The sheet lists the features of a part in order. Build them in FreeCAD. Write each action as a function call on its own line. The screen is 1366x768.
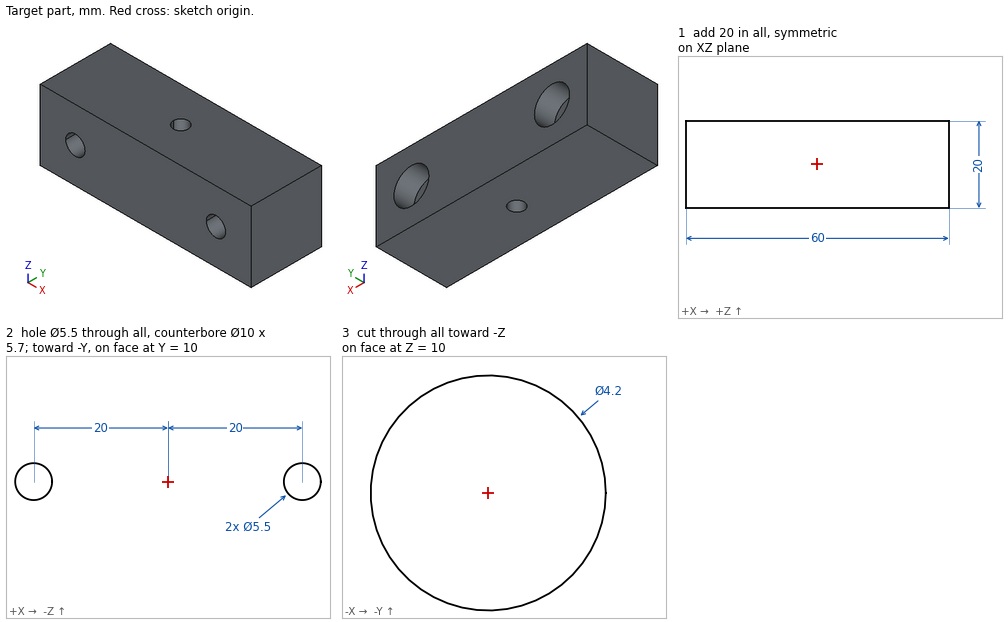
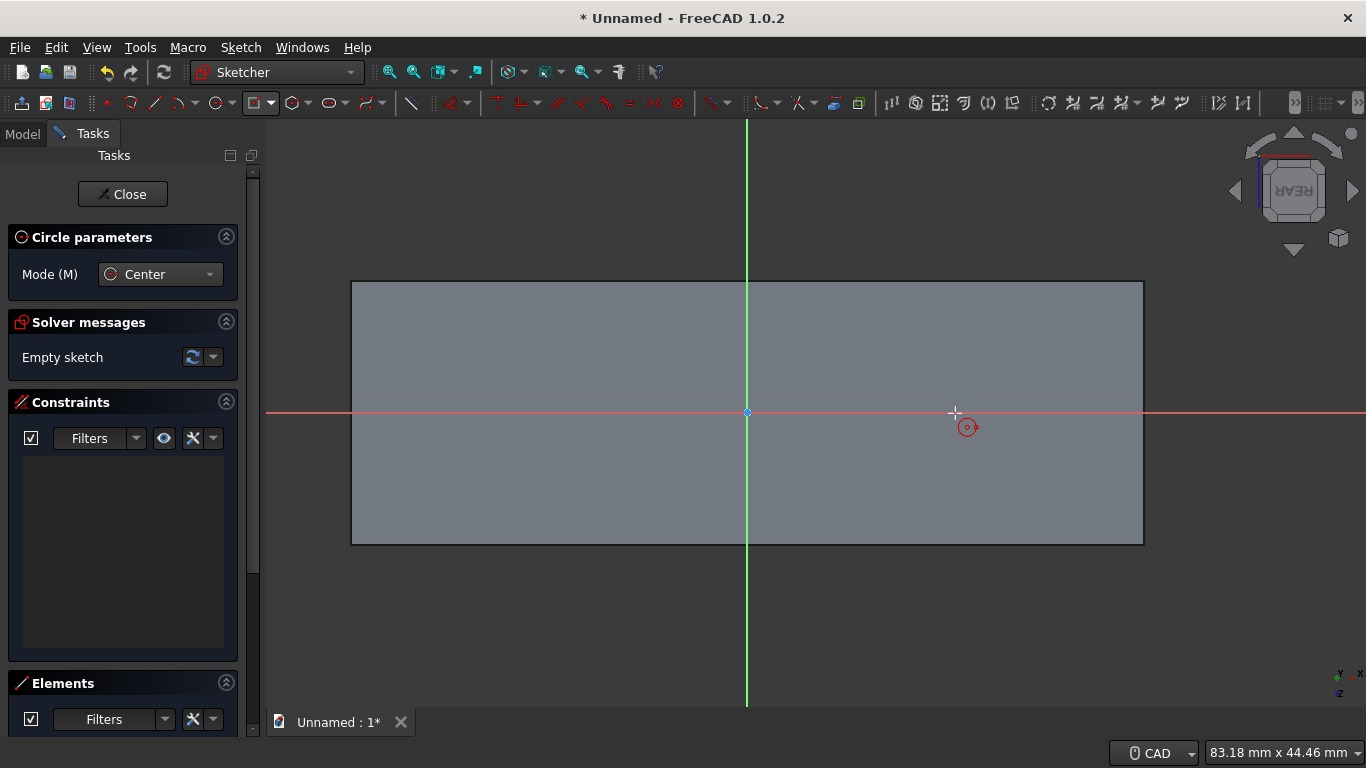
click(1012, 413)
move(1038, 387)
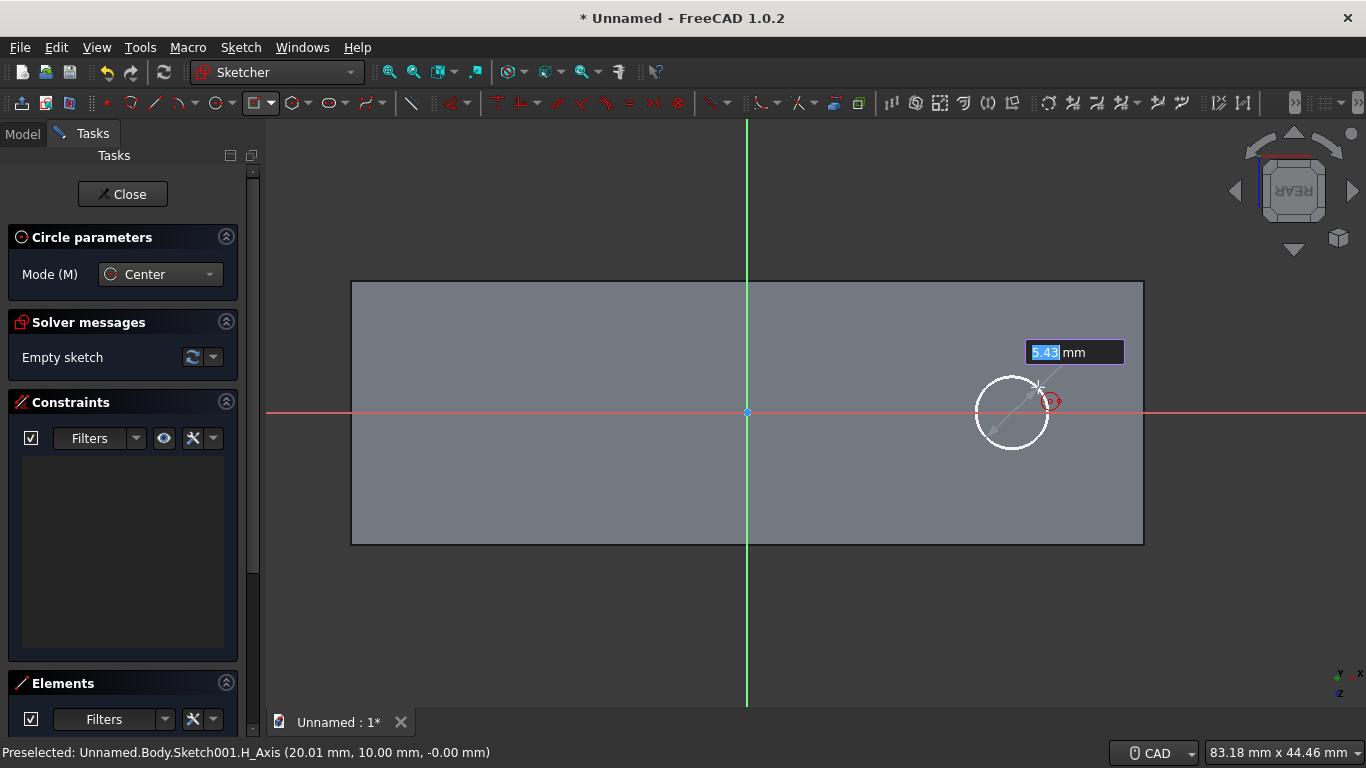
text(5.5)
key(Return)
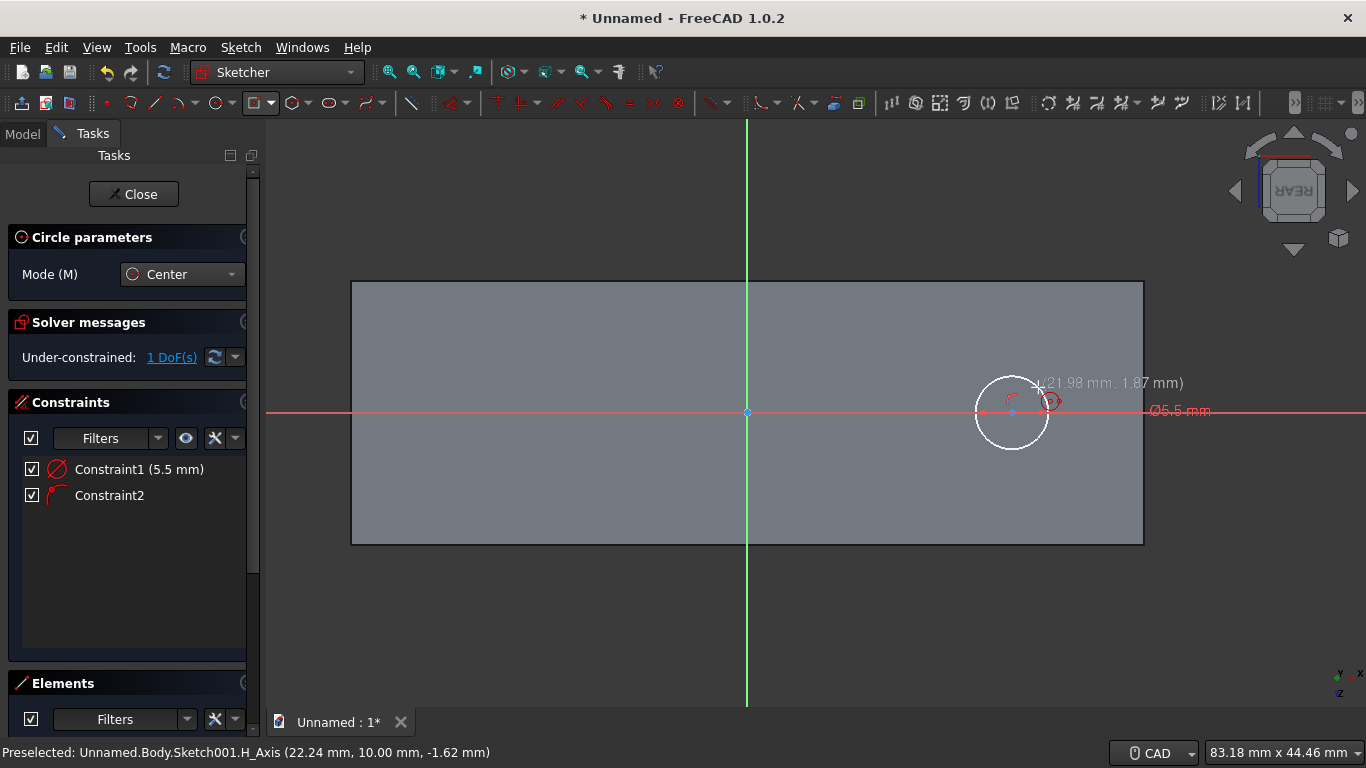
click(483, 413)
move(509, 387)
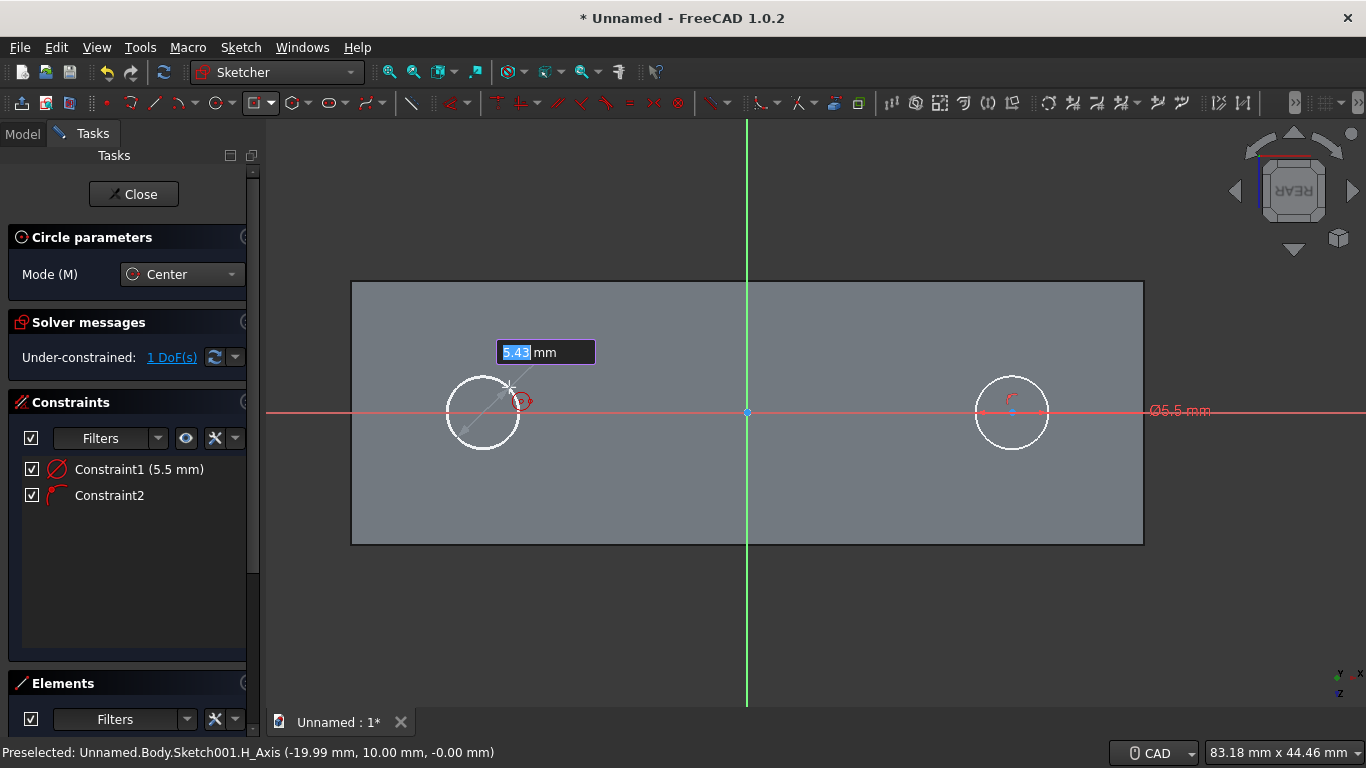
text(5.5)
key(Return)
key(Escape)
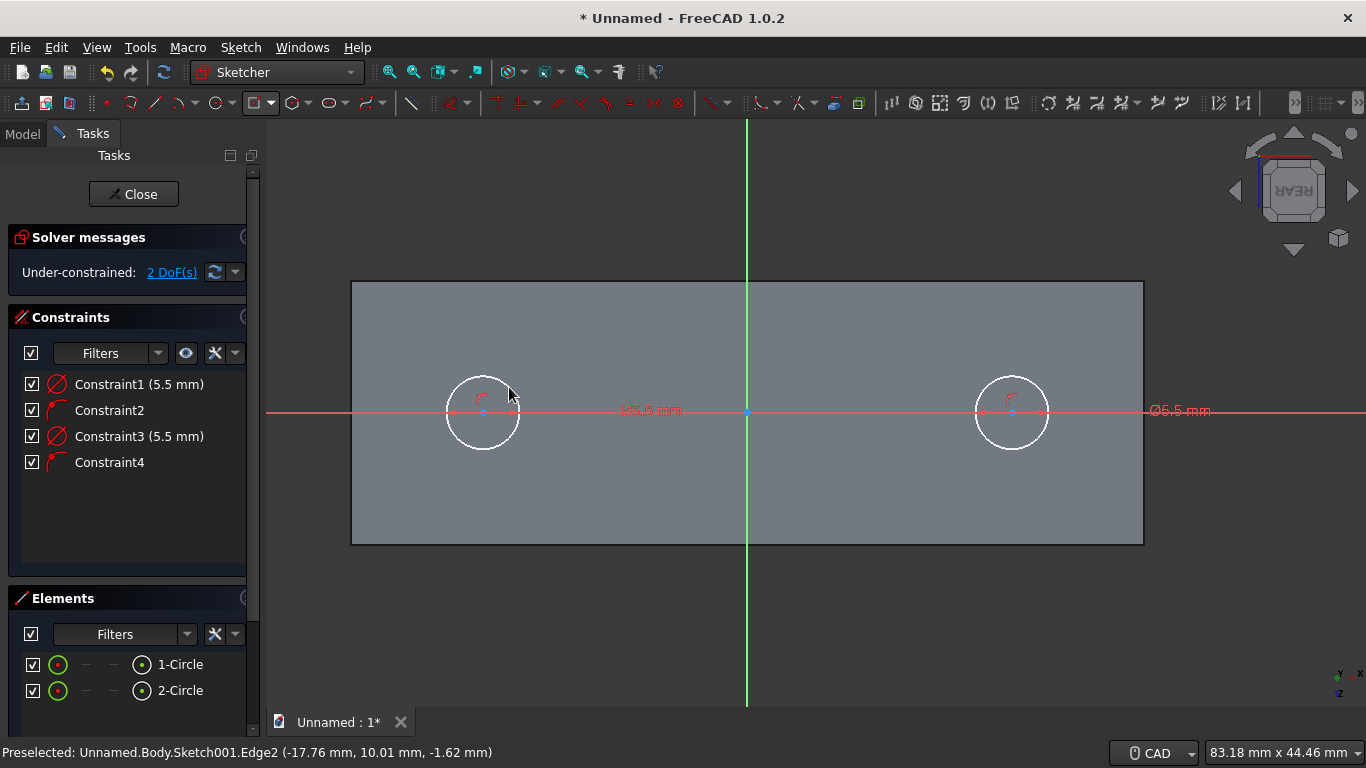
key(d)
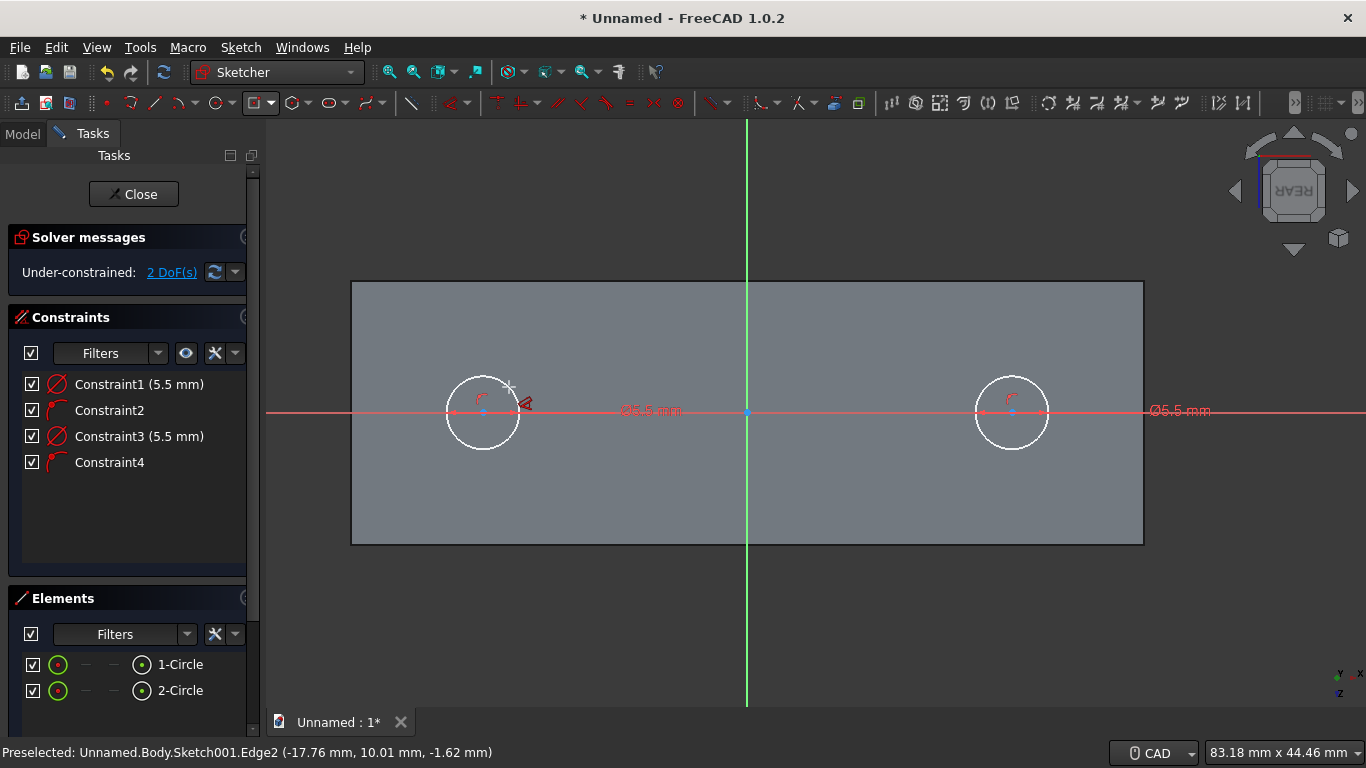
click(1012, 413)
click(880, 447)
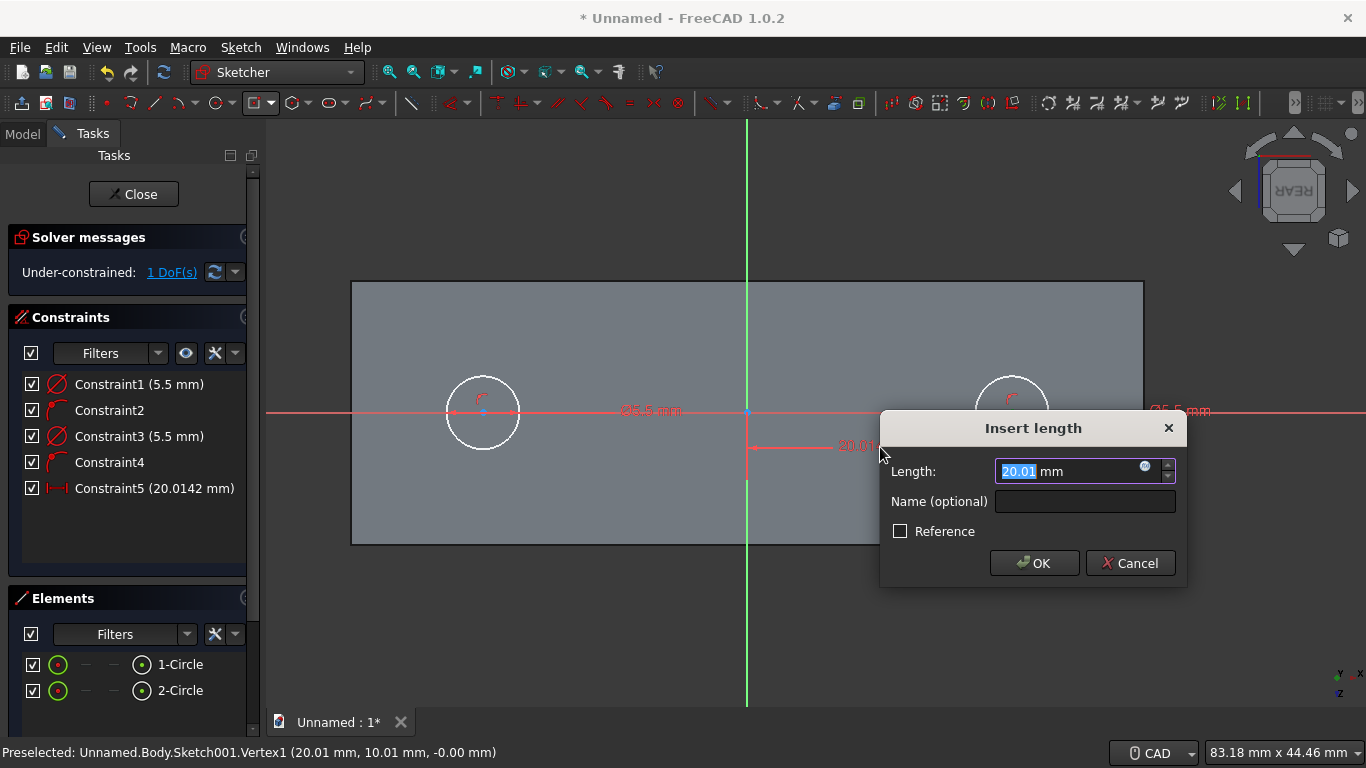
text(20)
key(Return)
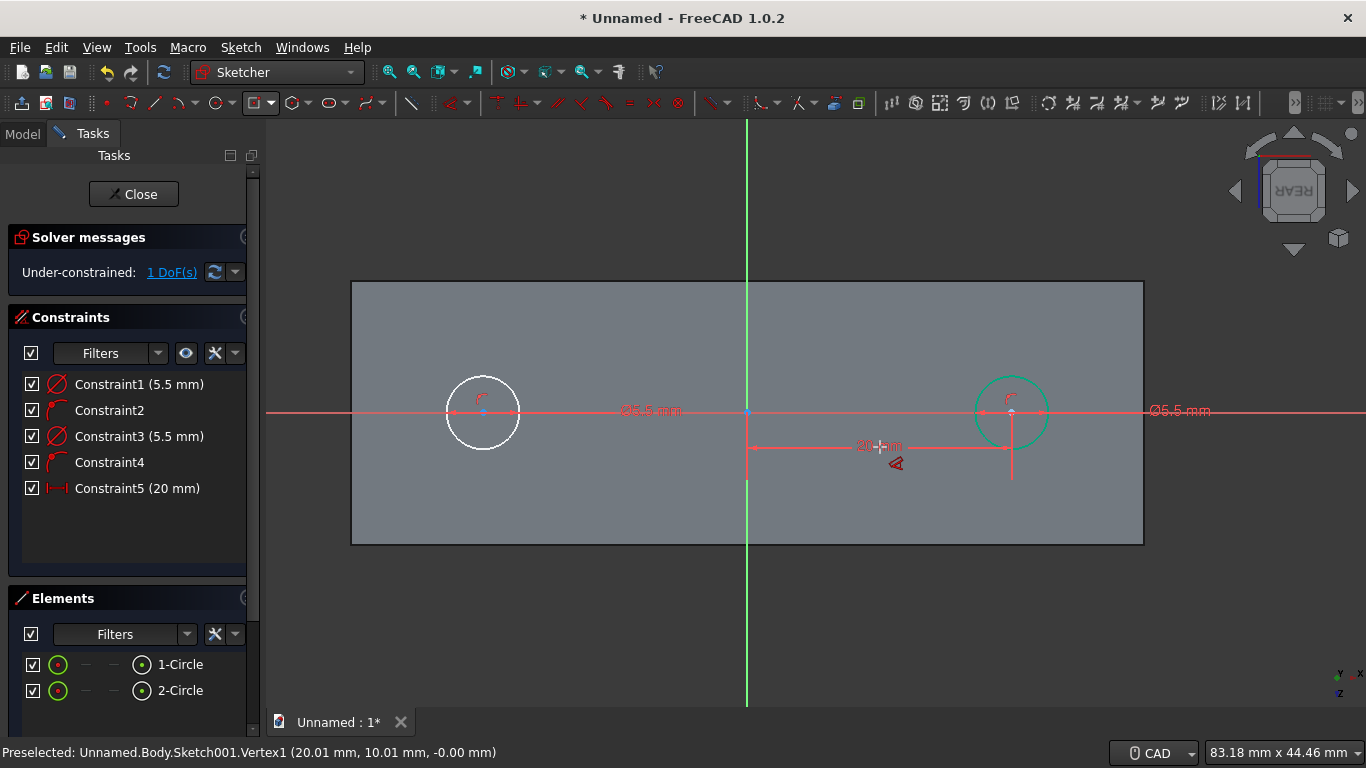
click(483, 413)
click(615, 447)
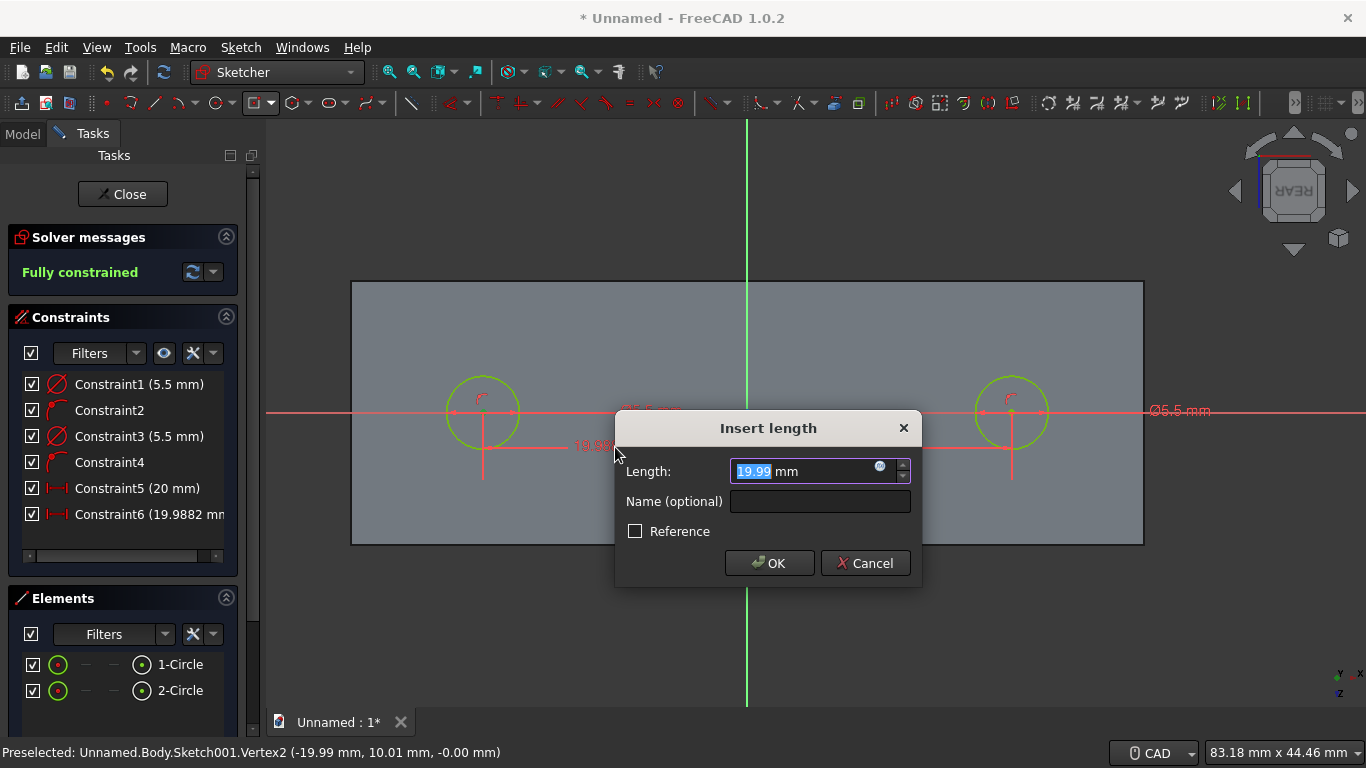
text(20)
key(Return)
key(Escape)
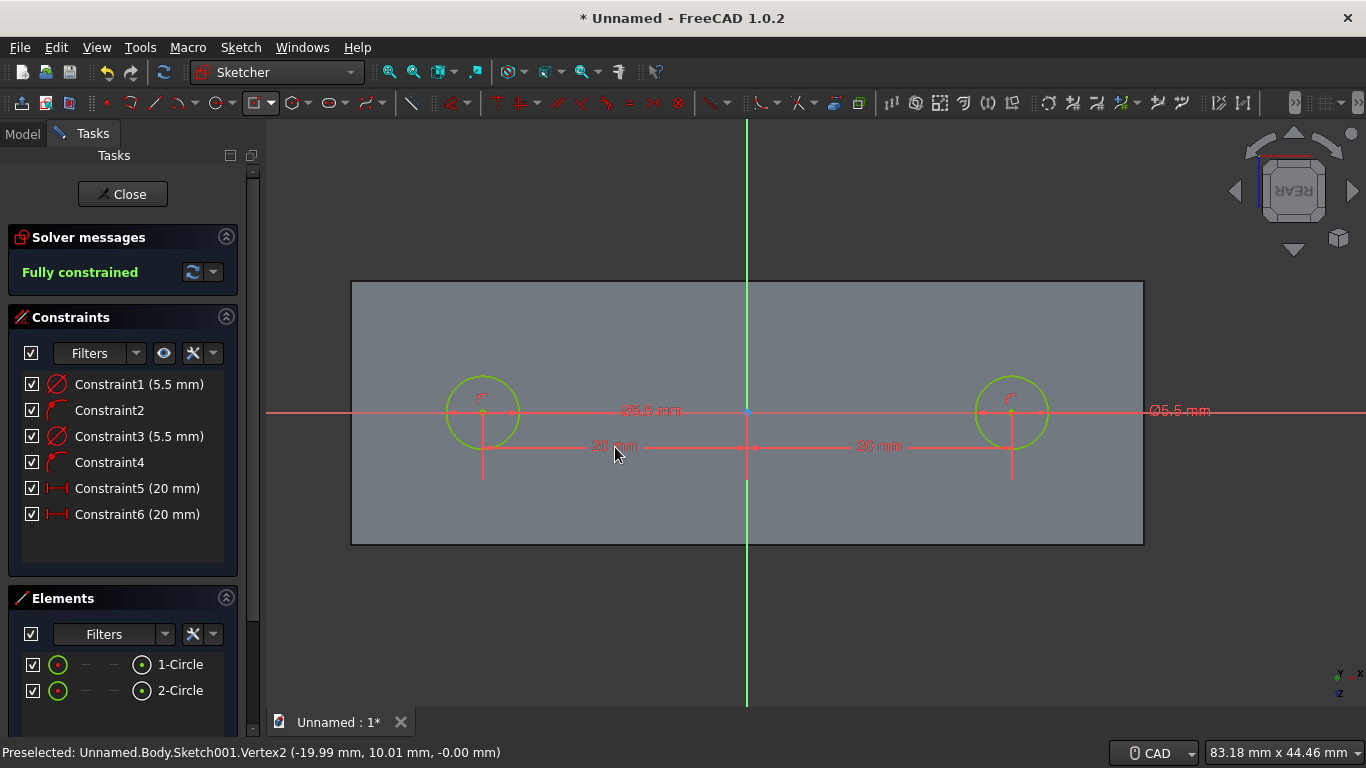
click(123, 194)